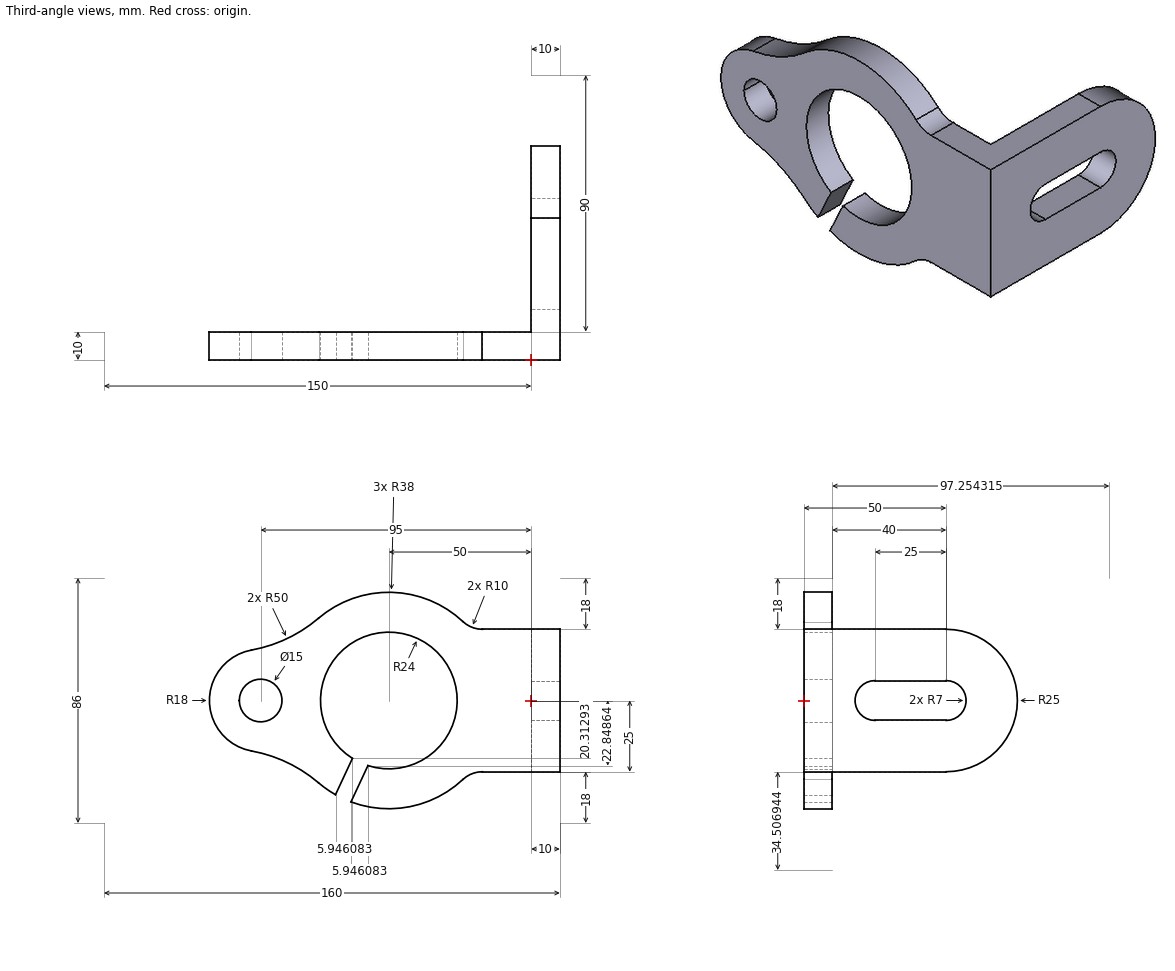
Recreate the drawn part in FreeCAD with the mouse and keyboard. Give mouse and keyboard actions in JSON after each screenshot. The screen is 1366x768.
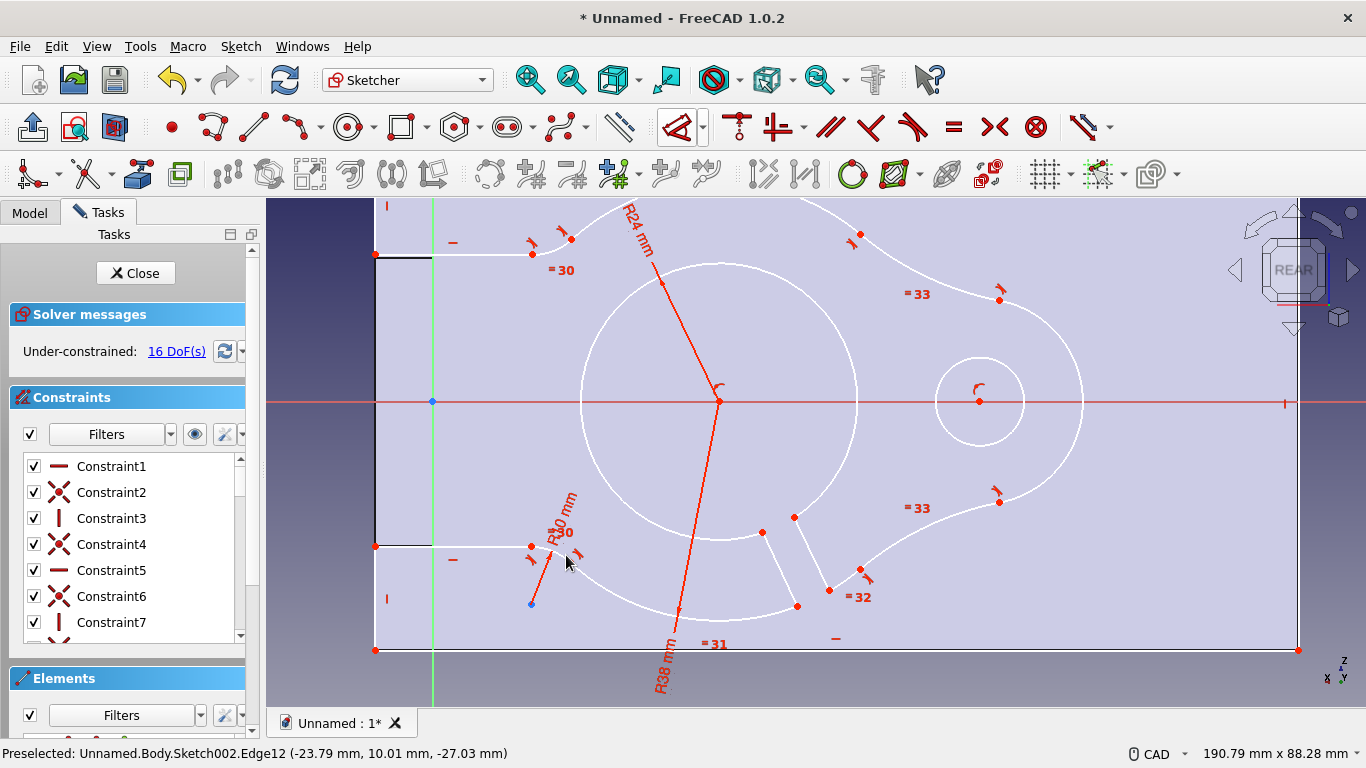
{"action": "left_click", "coordinate": [898, 261]}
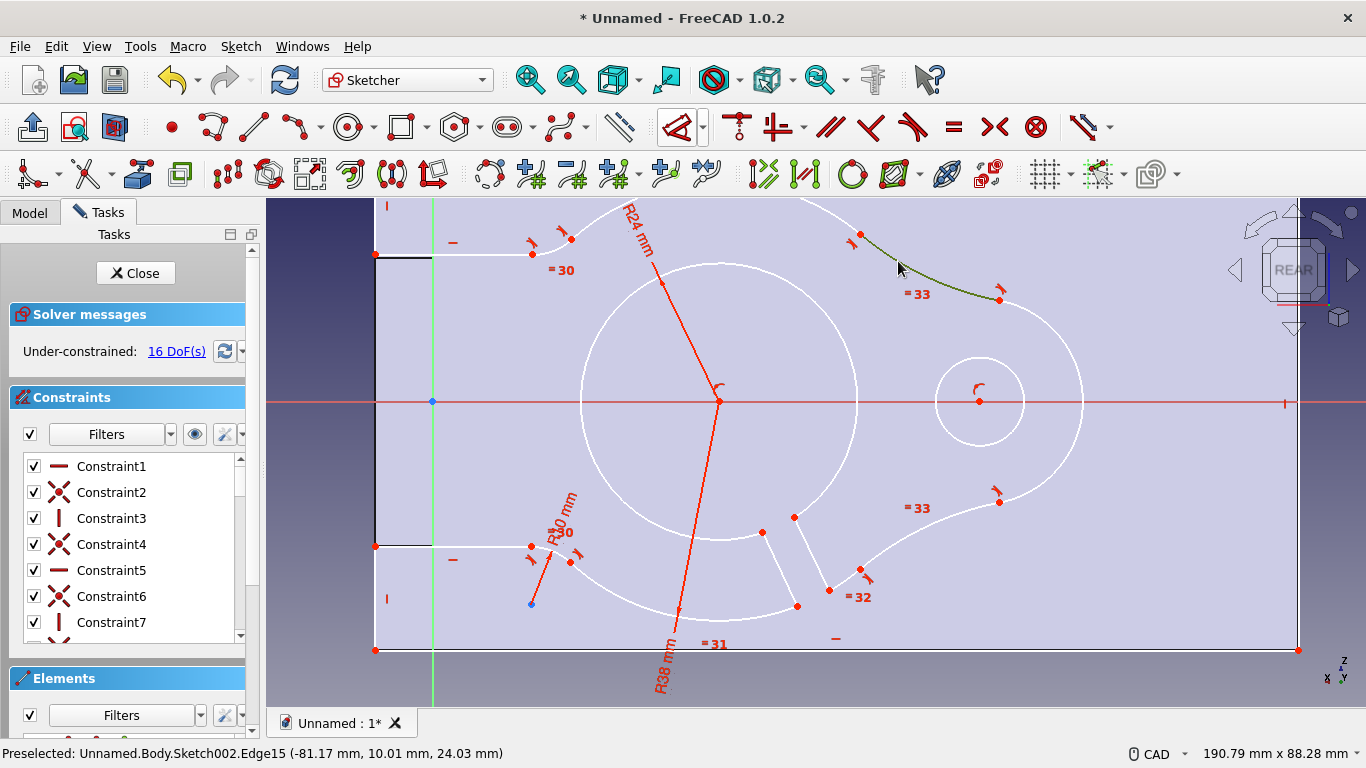
{"action": "key", "text": "k r"}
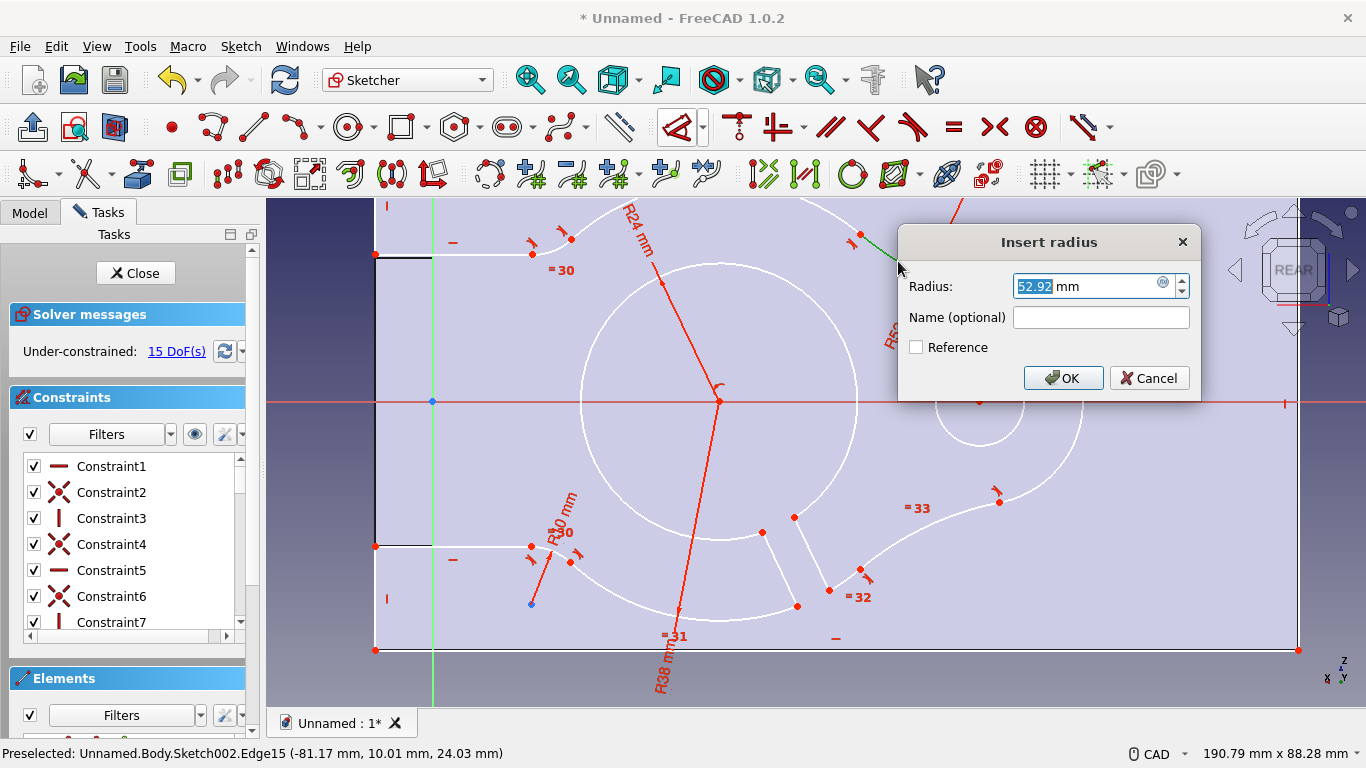
{"action": "type", "text": "50"}
{"action": "key", "text": "Return"}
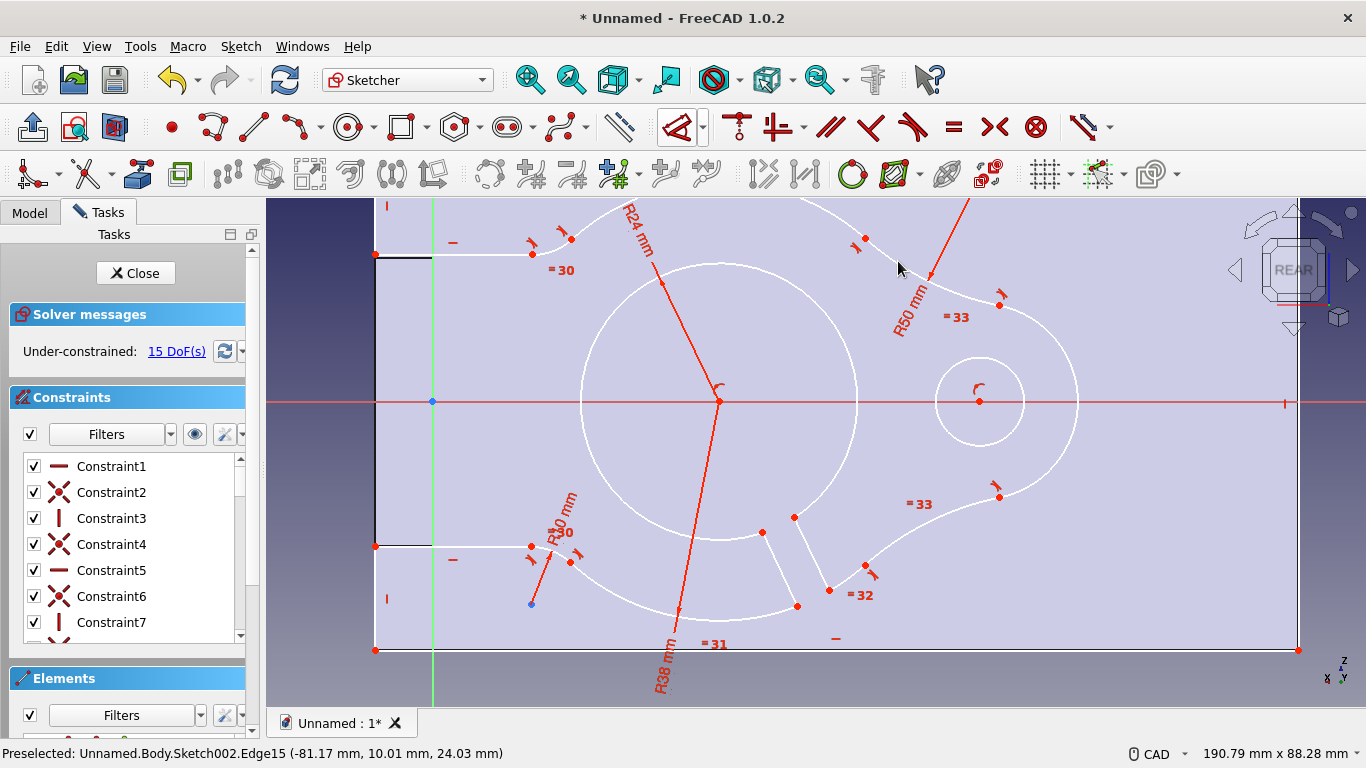
{"action": "left_click", "coordinate": [1064, 453]}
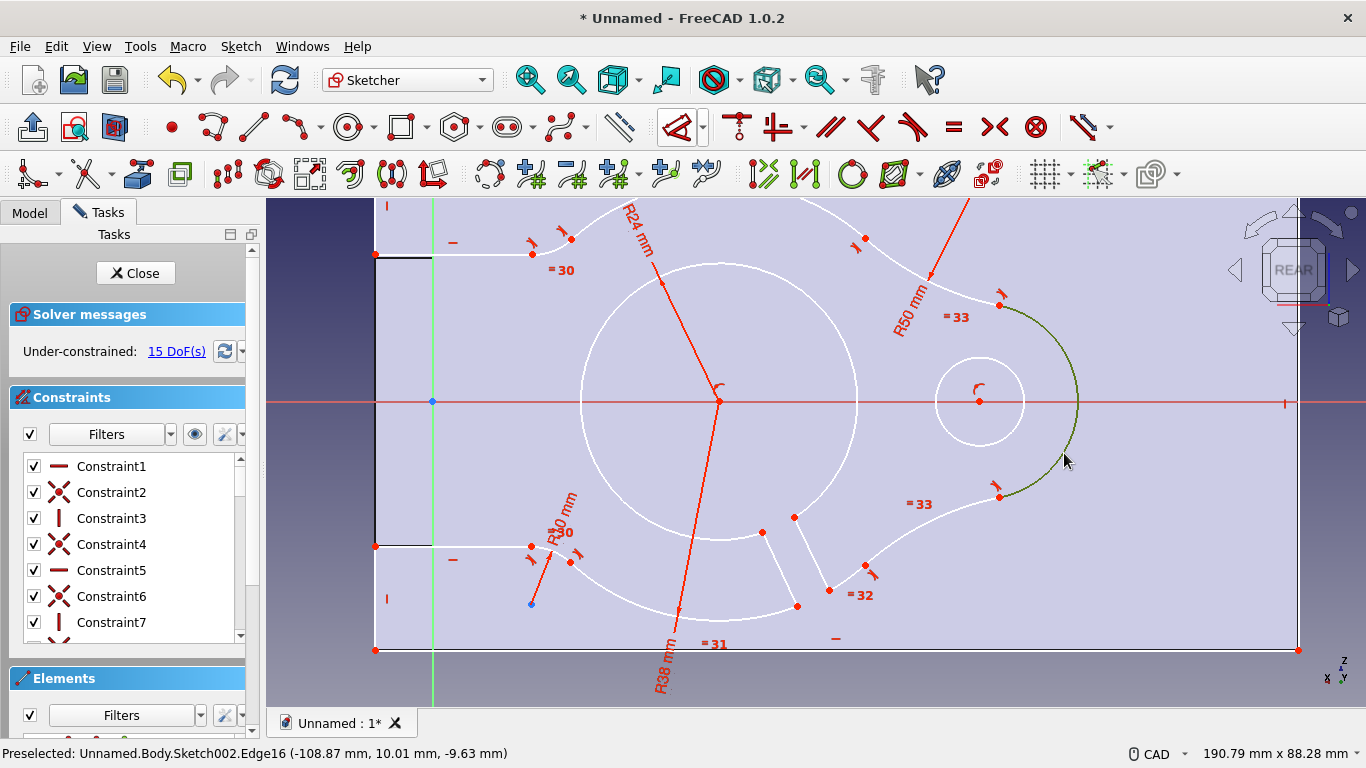
{"action": "left_click", "coordinate": [702, 128]}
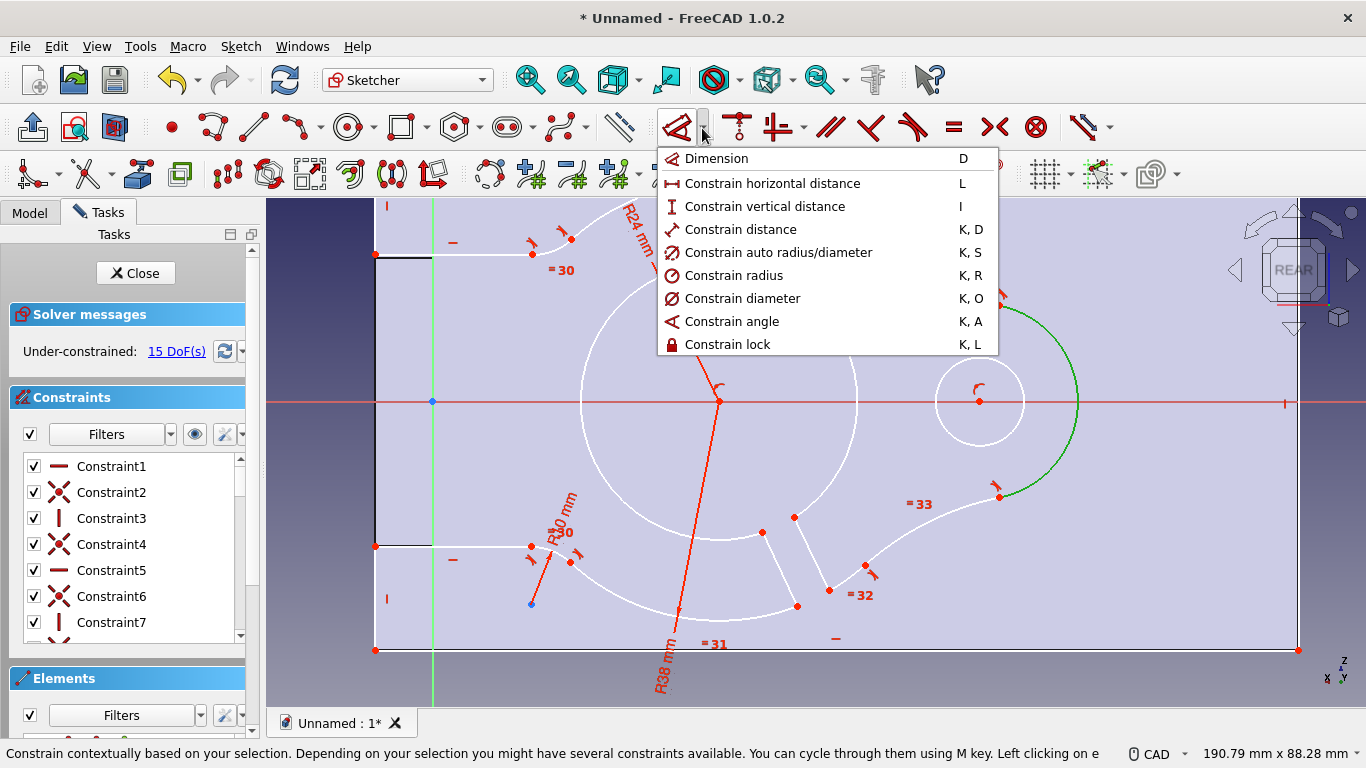
{"action": "left_click", "coordinate": [828, 276]}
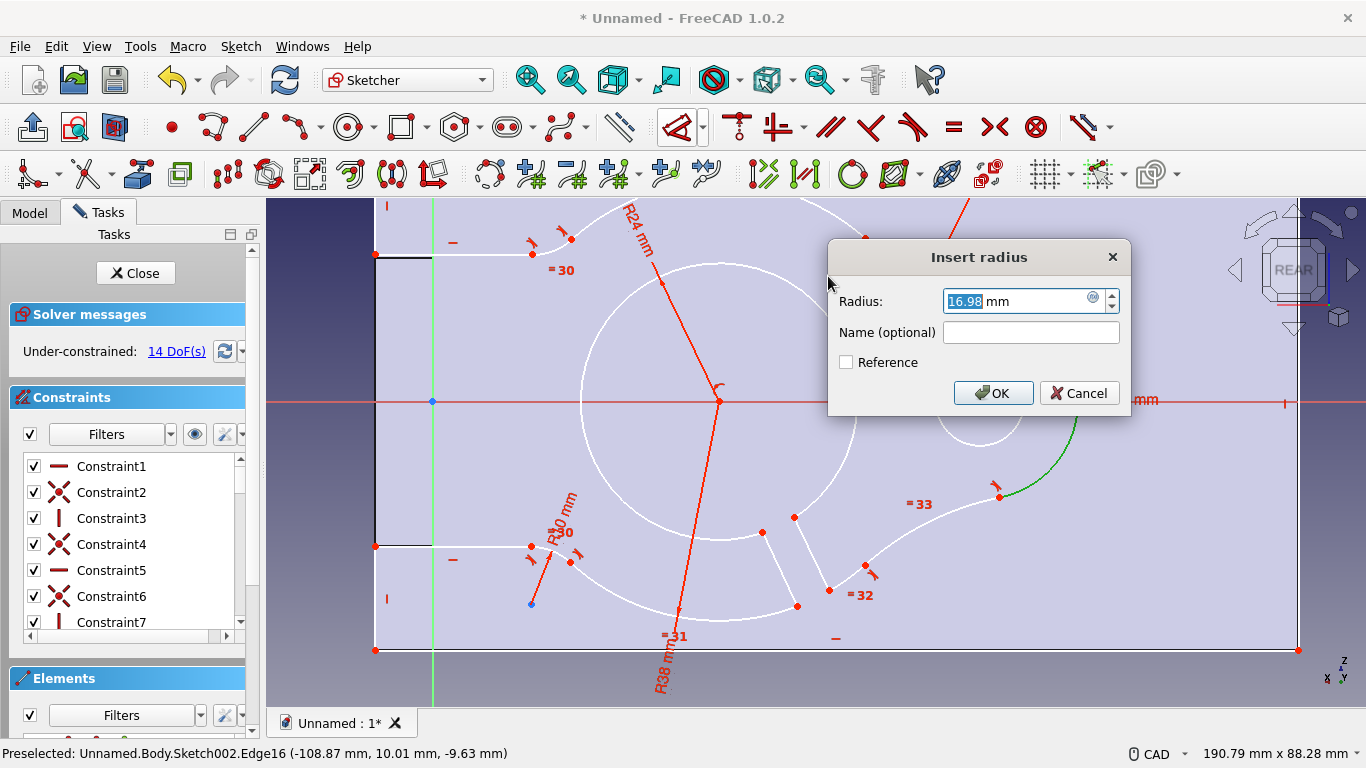
{"action": "type", "text": "18"}
{"action": "key", "text": "Return"}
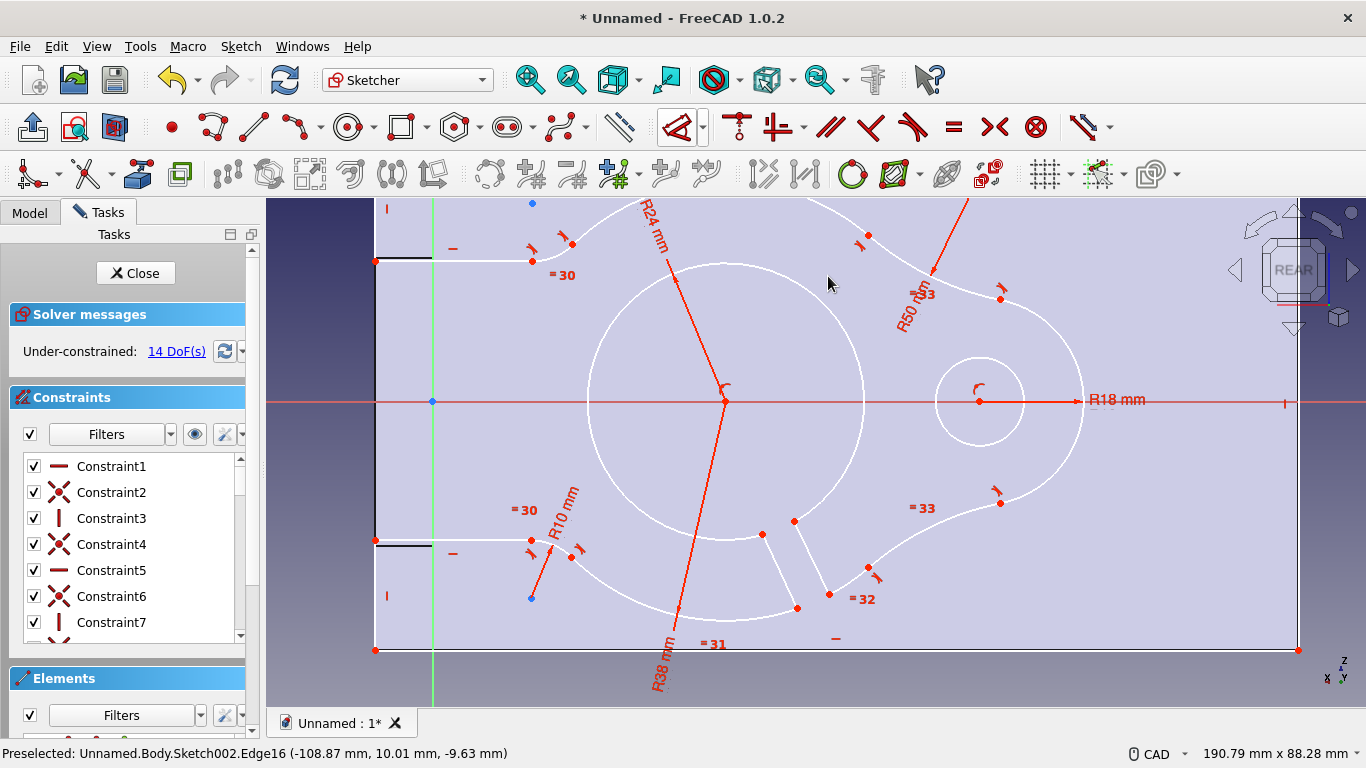
{"action": "left_click", "coordinate": [1011, 370]}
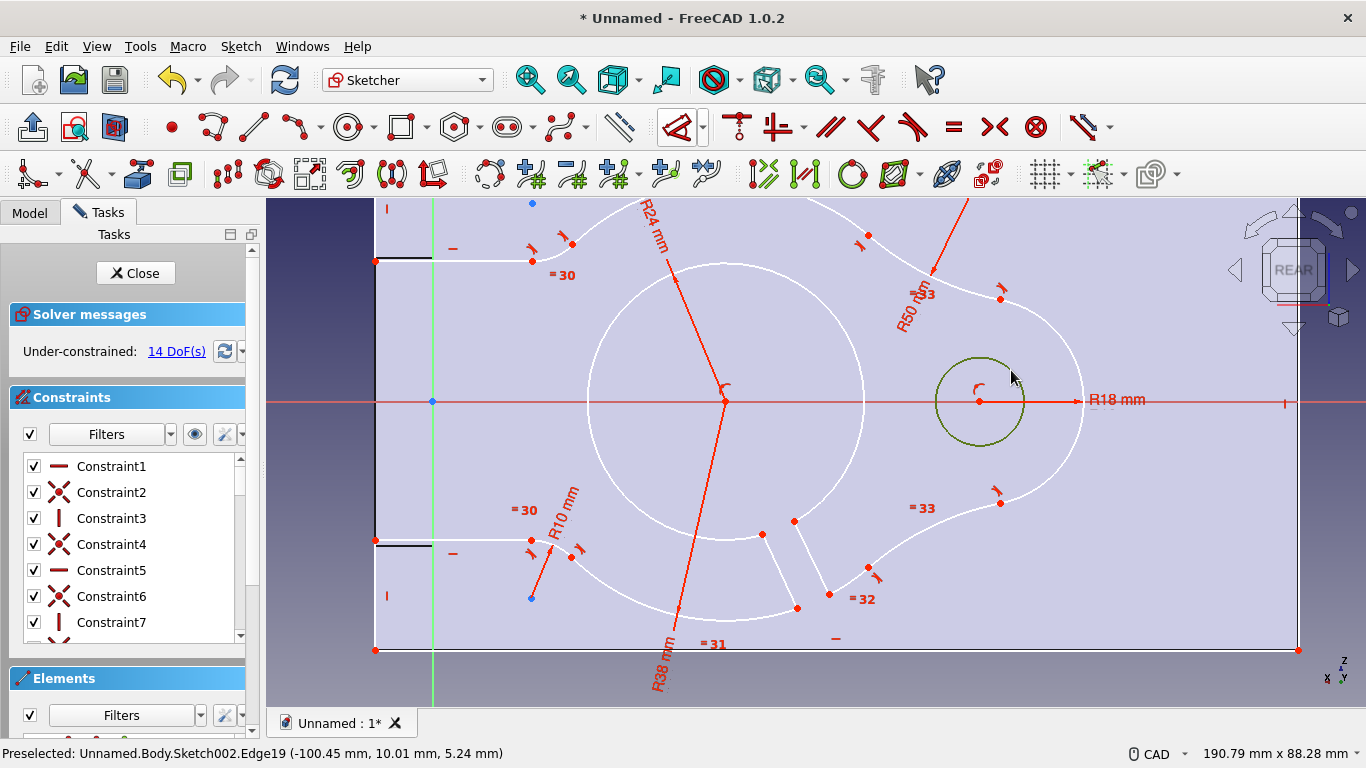
{"action": "key", "text": "k o"}